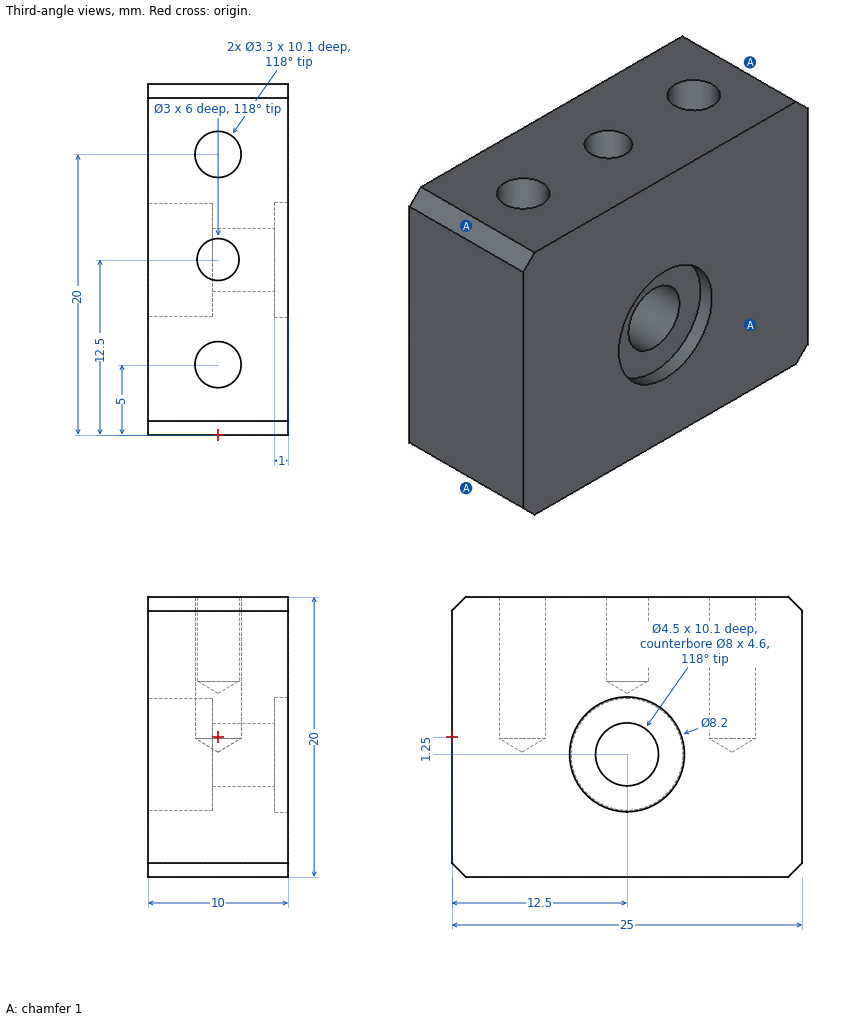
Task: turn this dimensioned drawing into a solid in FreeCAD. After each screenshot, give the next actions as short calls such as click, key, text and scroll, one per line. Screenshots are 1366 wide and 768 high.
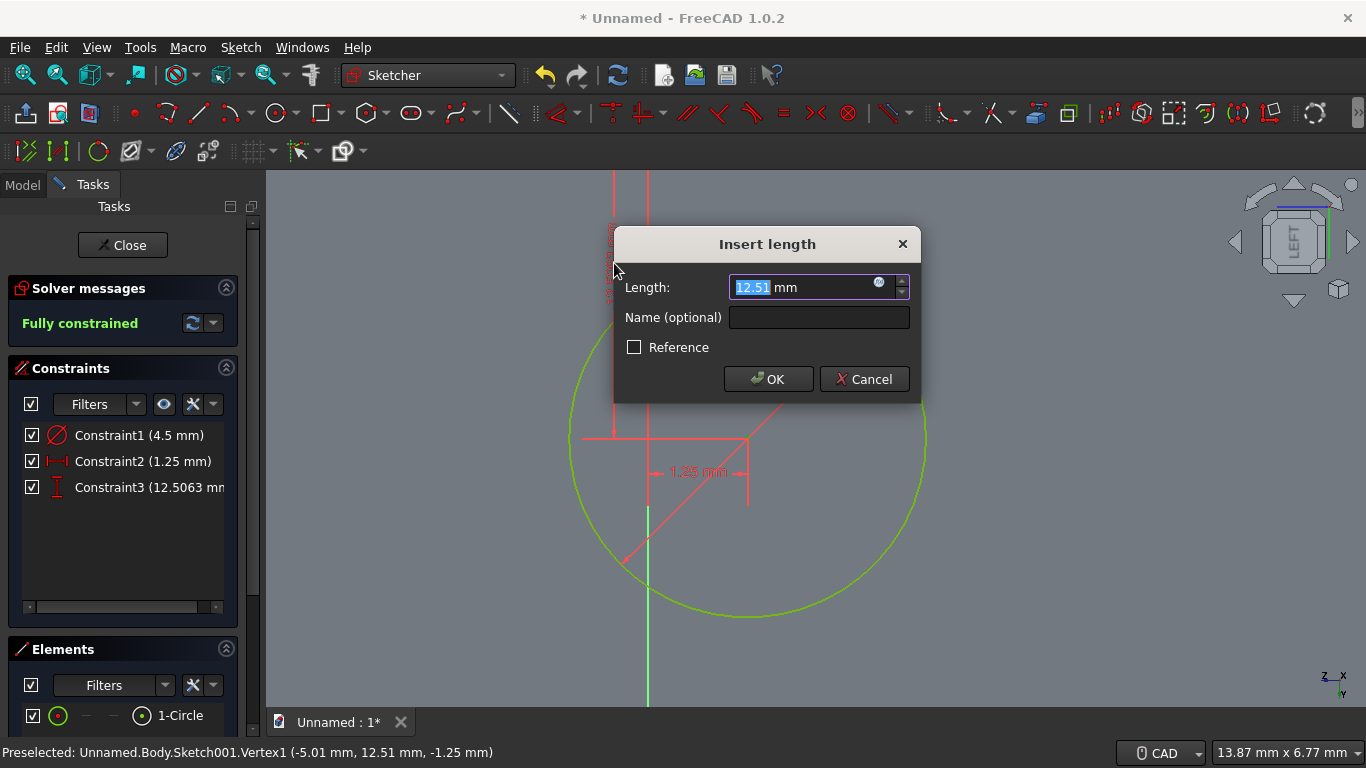
text(12.5)
key(Return)
key(Escape)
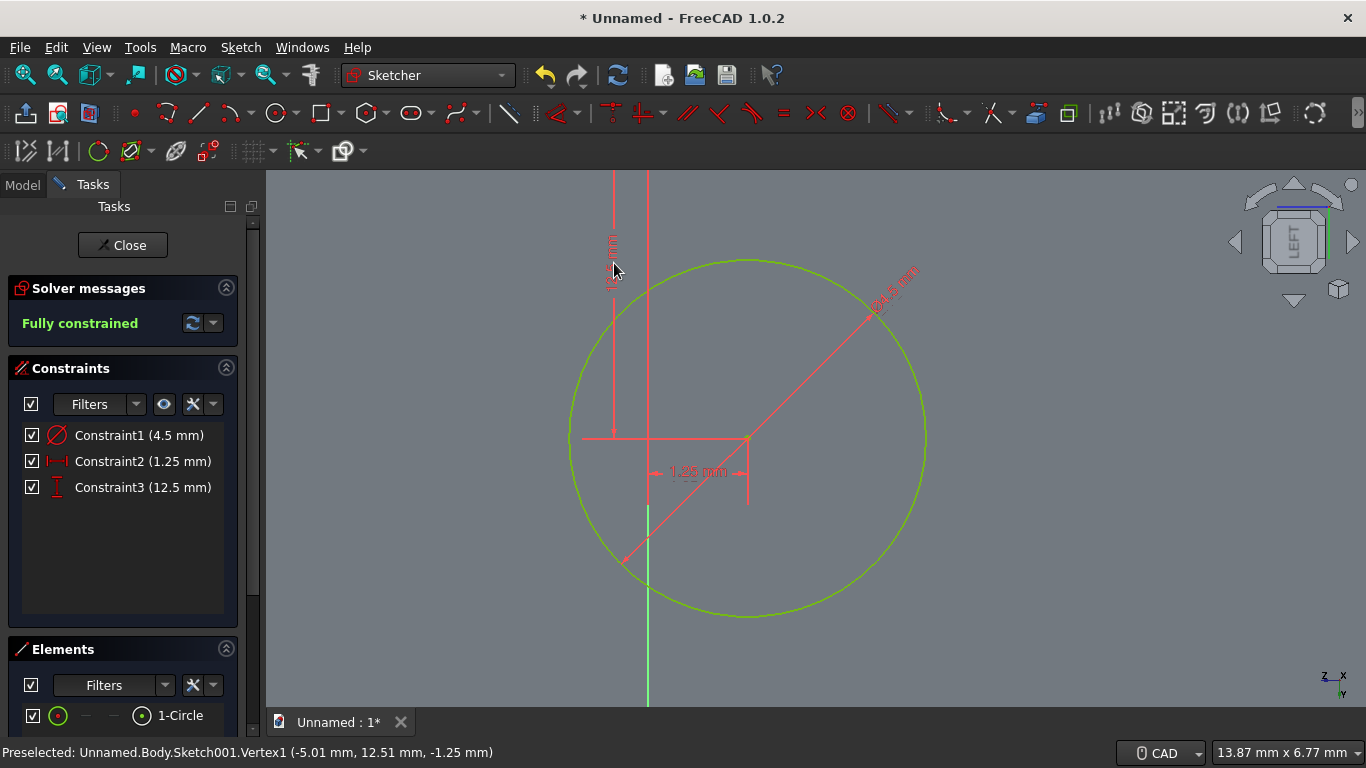
click(123, 245)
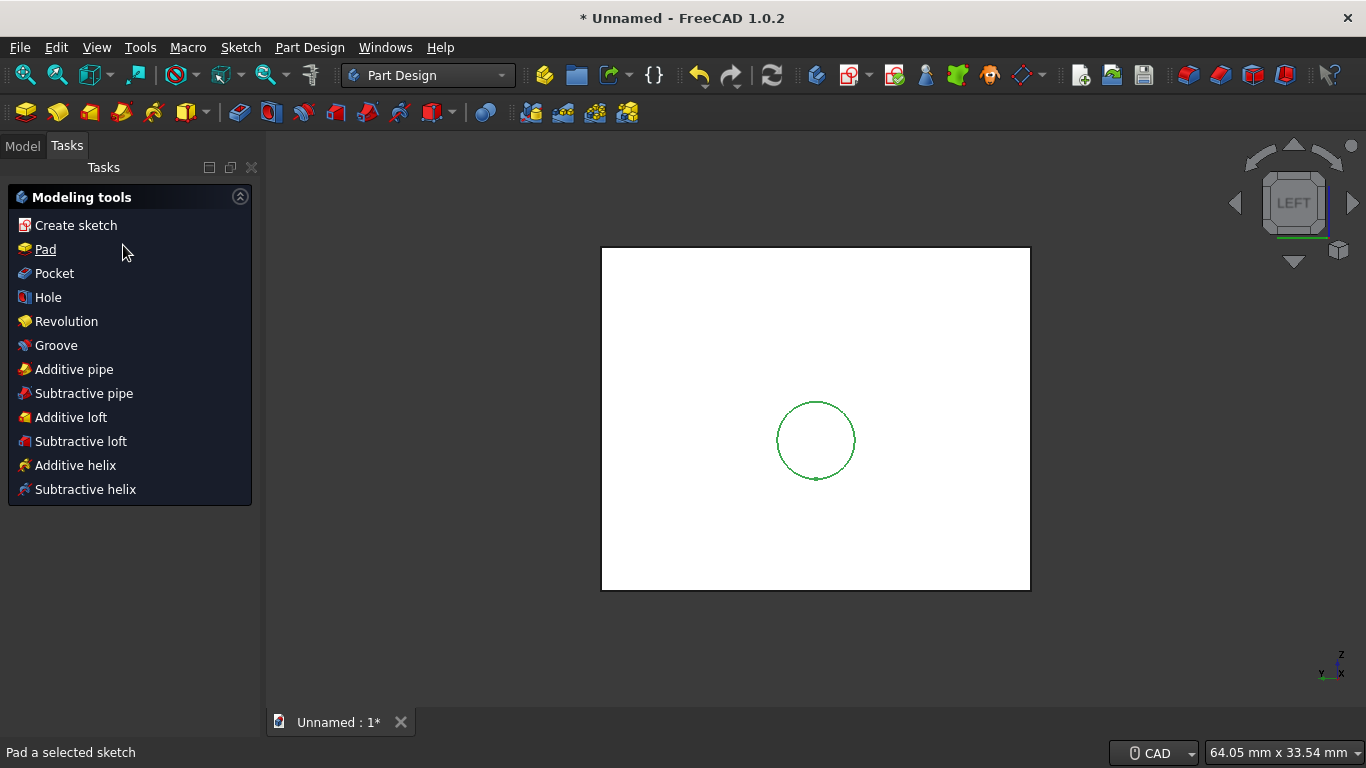
click(272, 112)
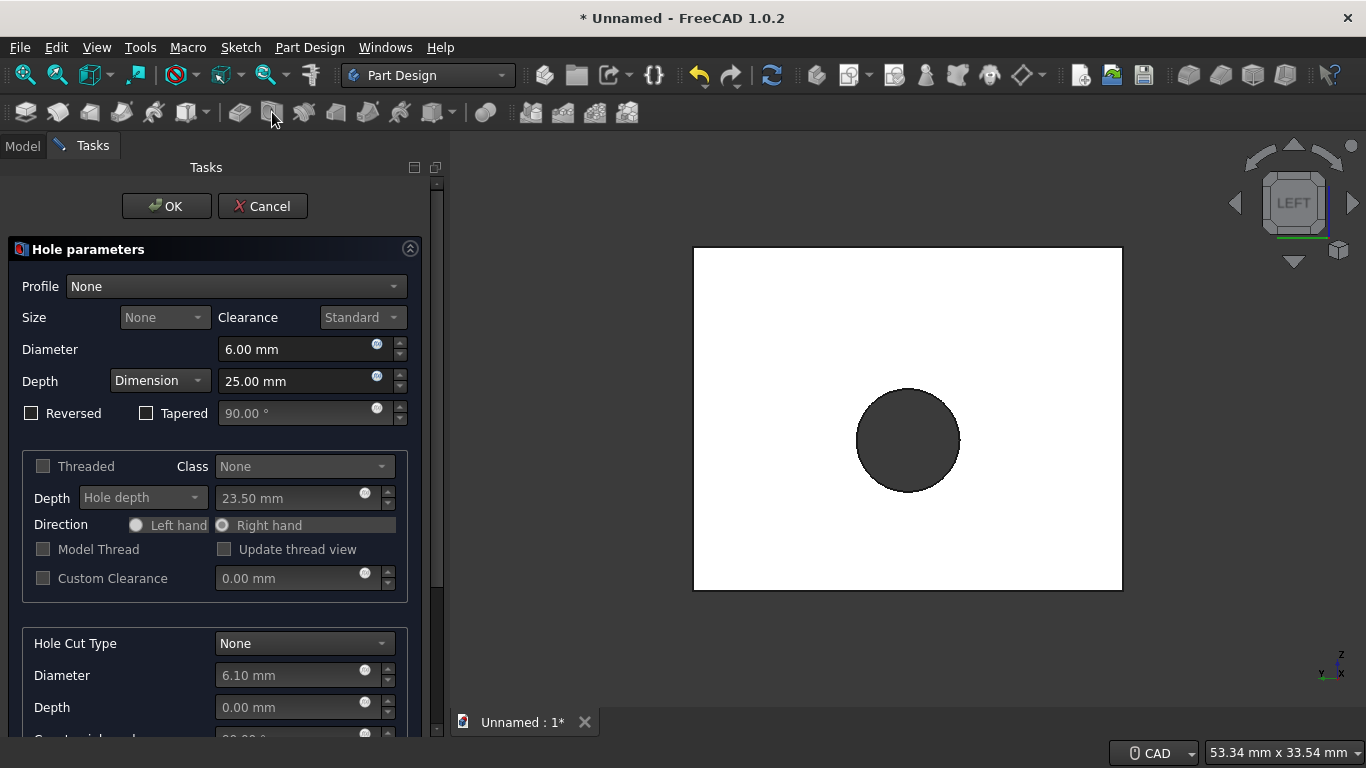
triple_click(305, 349)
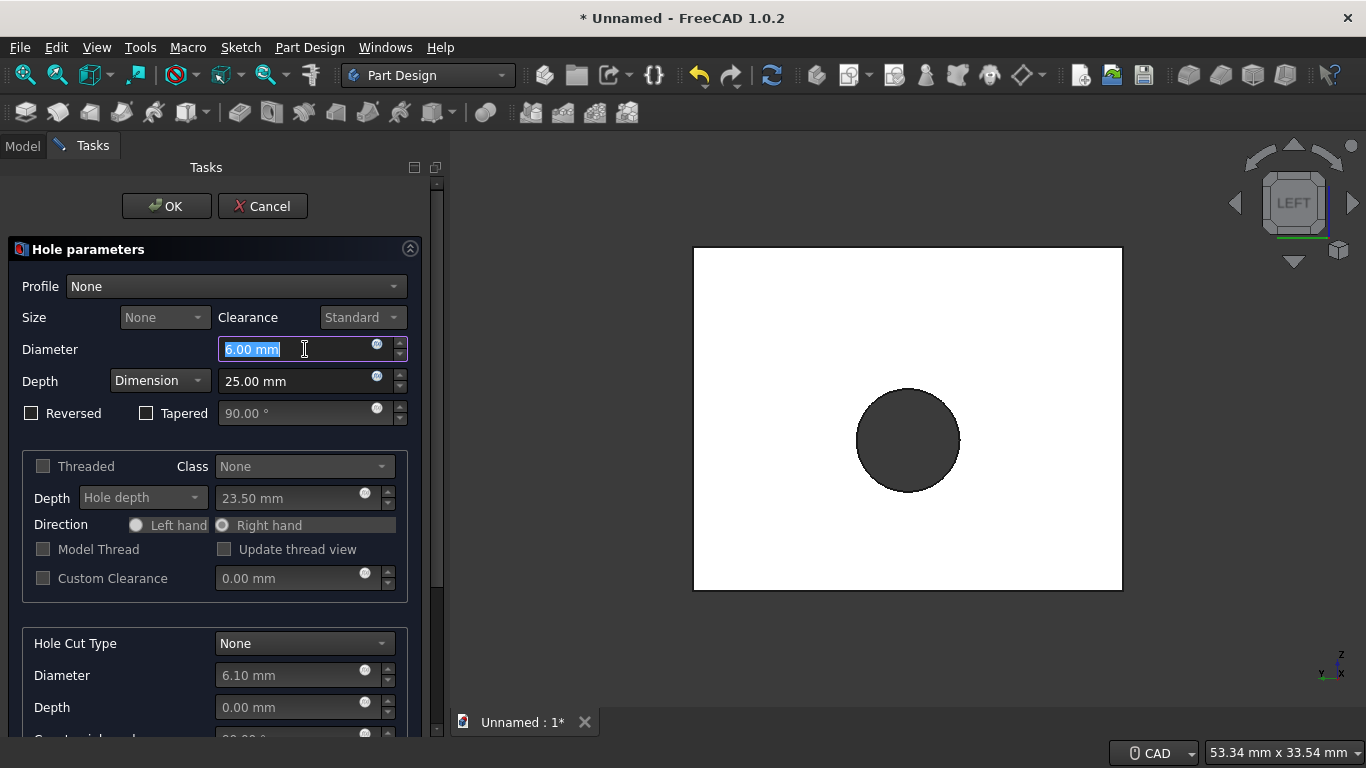
text(4.5)
key(Tab)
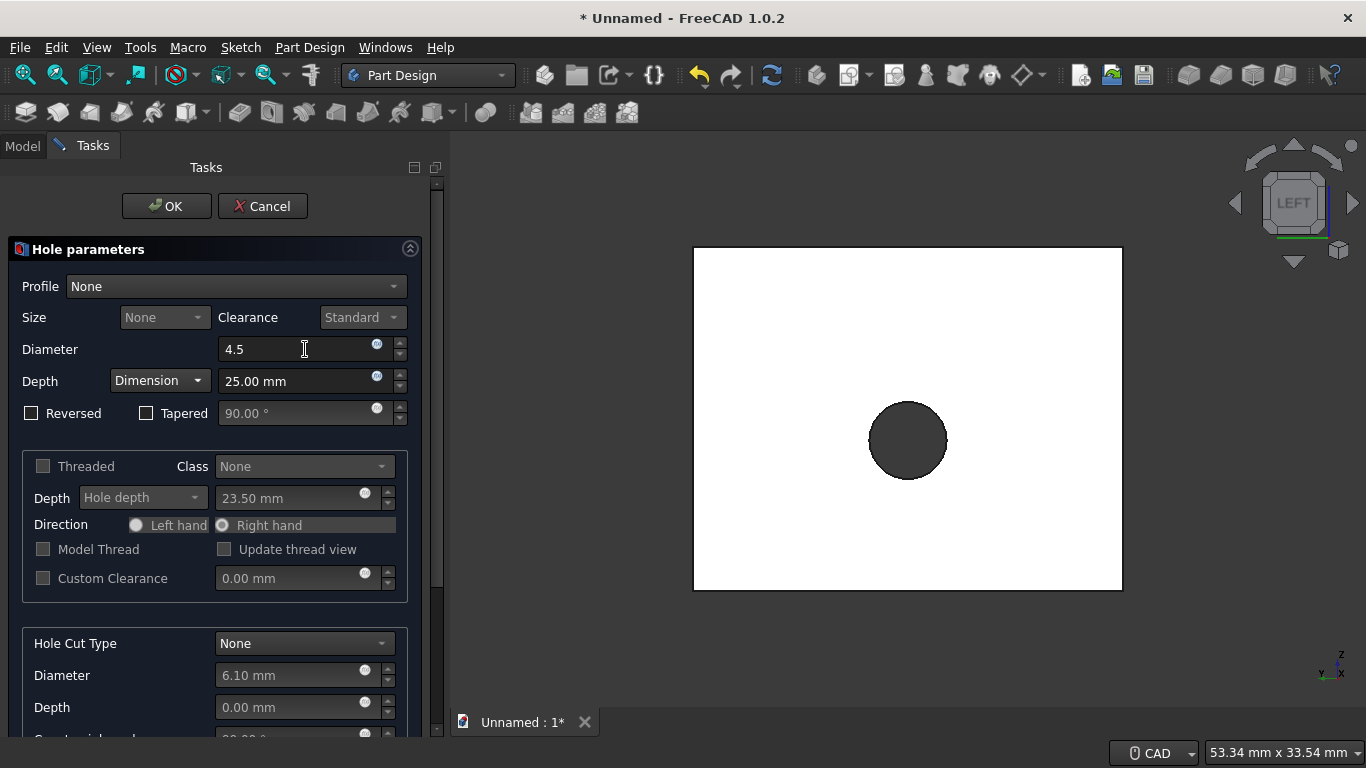
triple_click(305, 381)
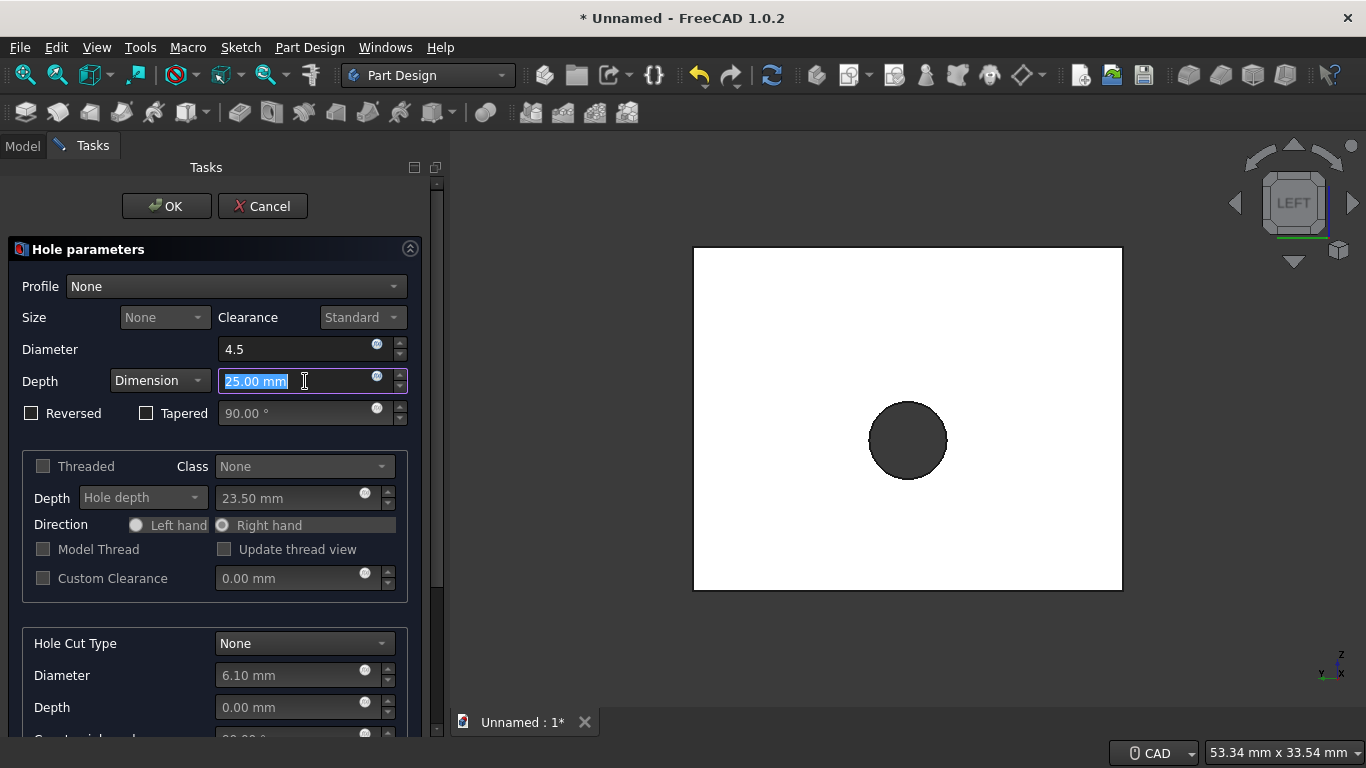
text(10.1)
key(Tab)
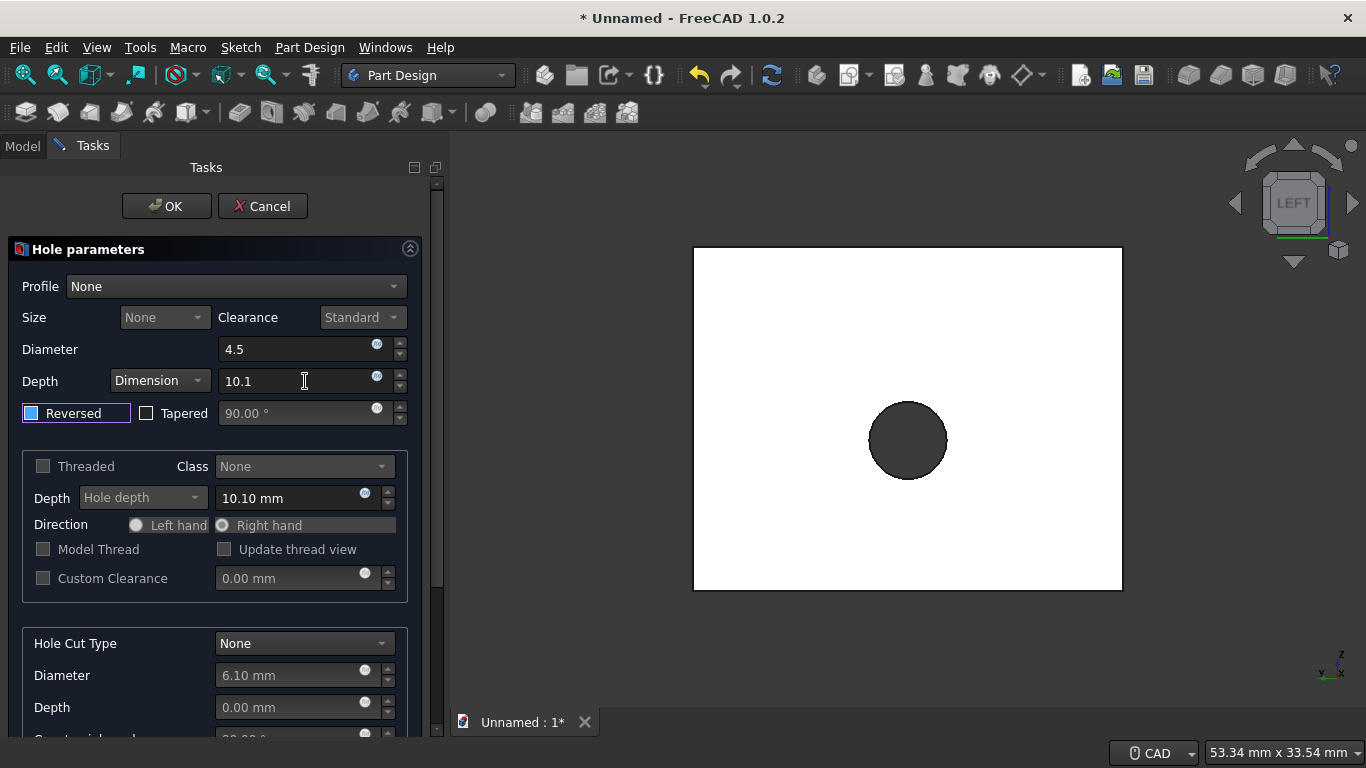
click(306, 644)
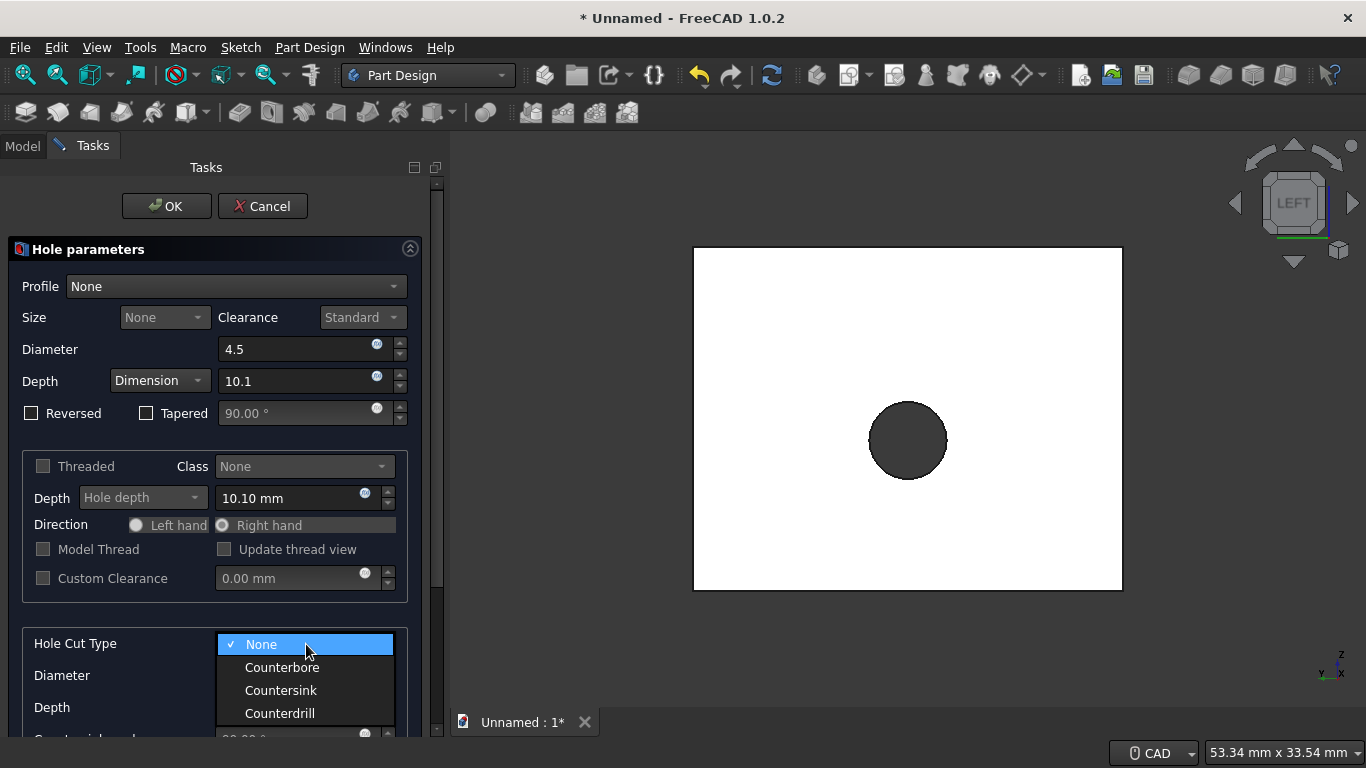
click(304, 668)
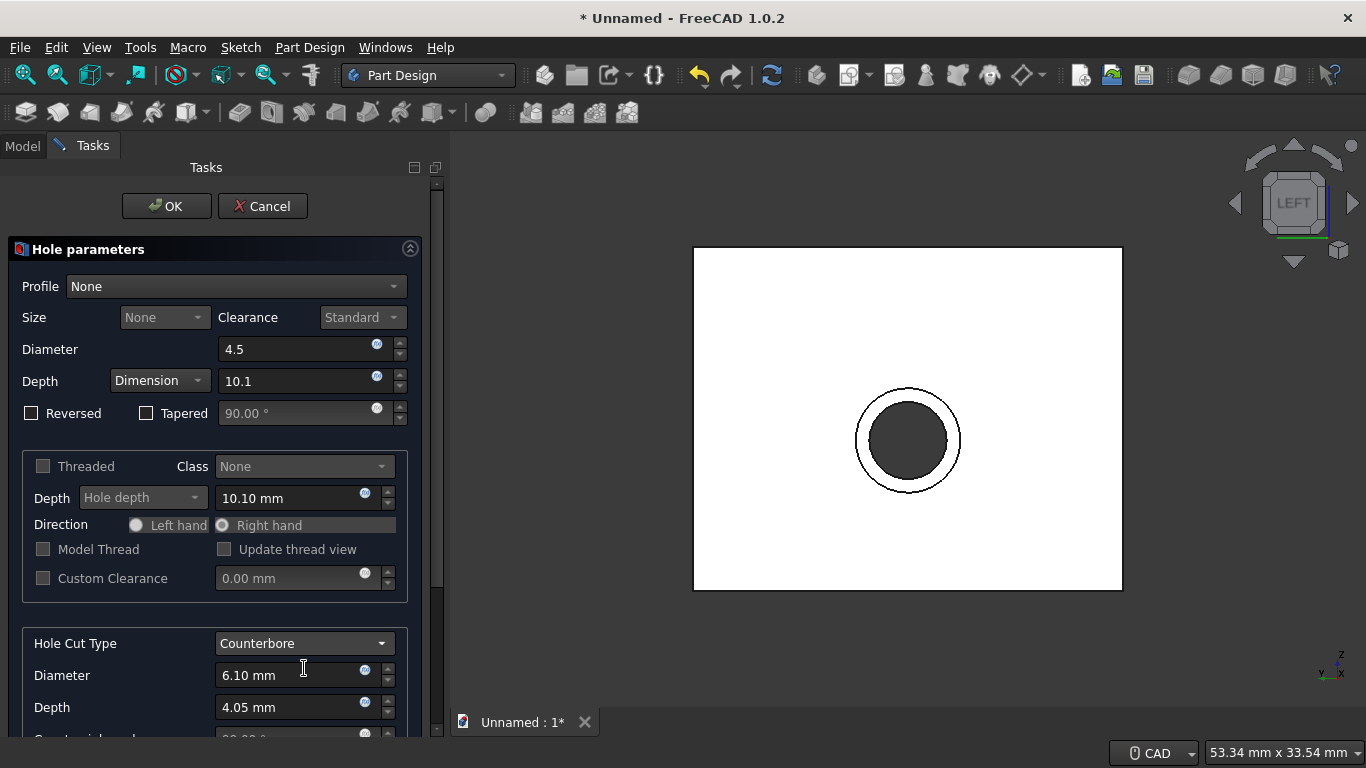
triple_click(298, 675)